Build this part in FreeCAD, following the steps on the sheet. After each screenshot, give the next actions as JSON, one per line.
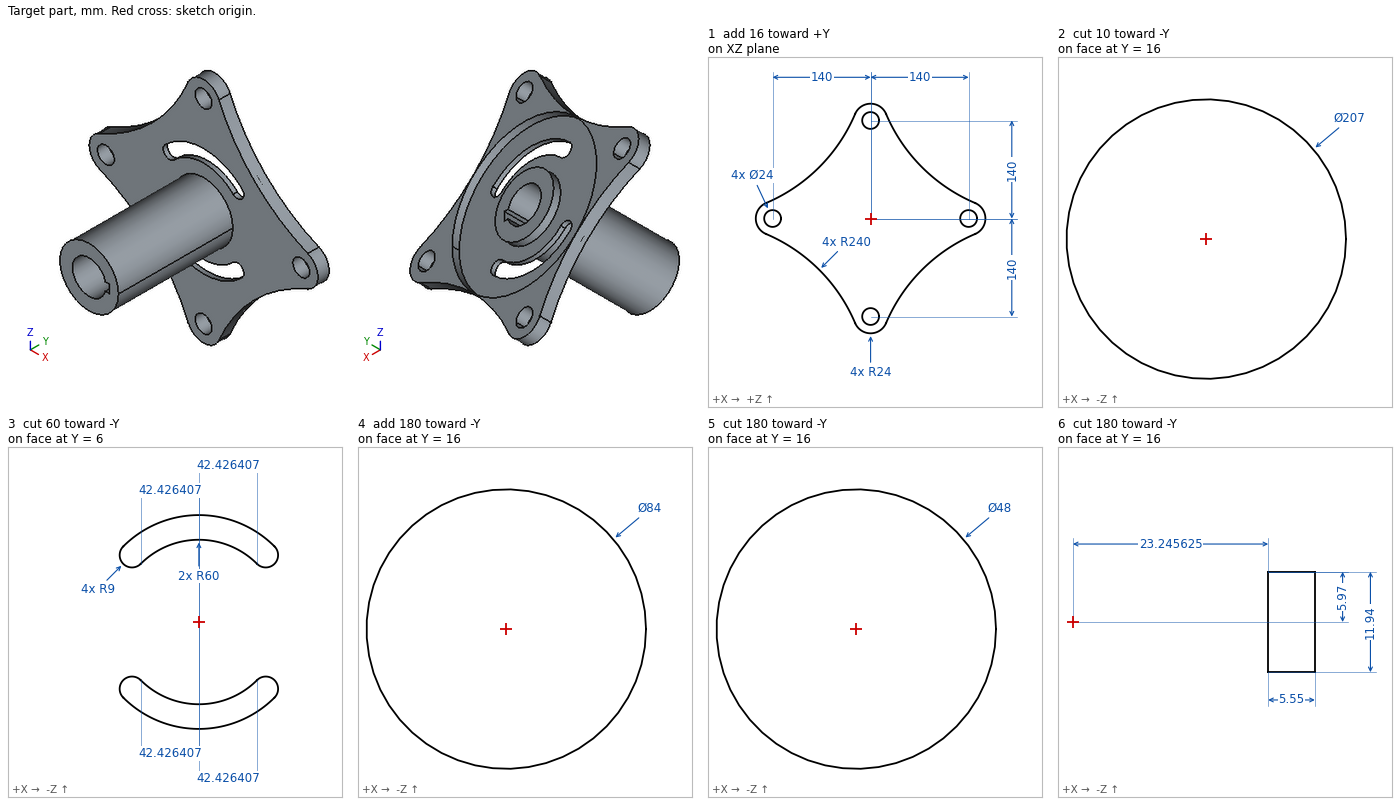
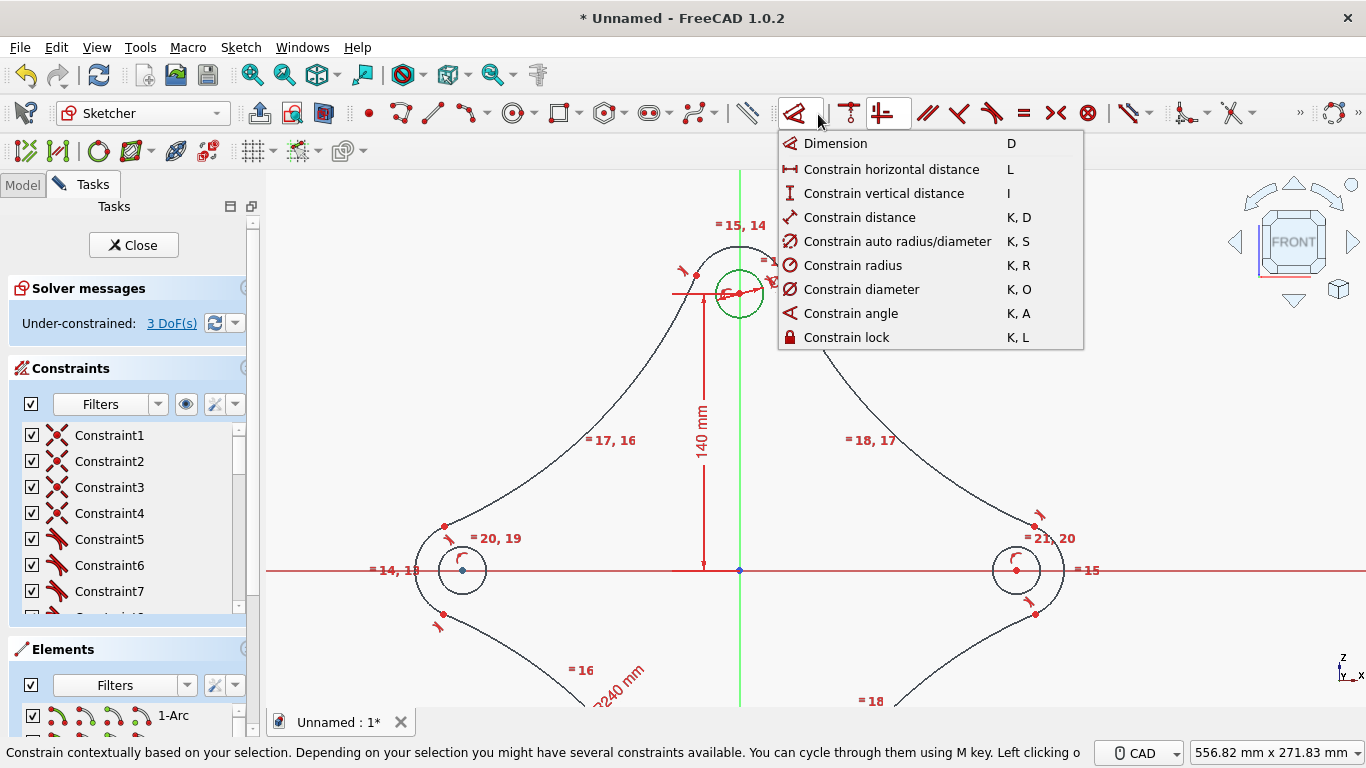
{"action": "left_click", "coordinate": [931, 169]}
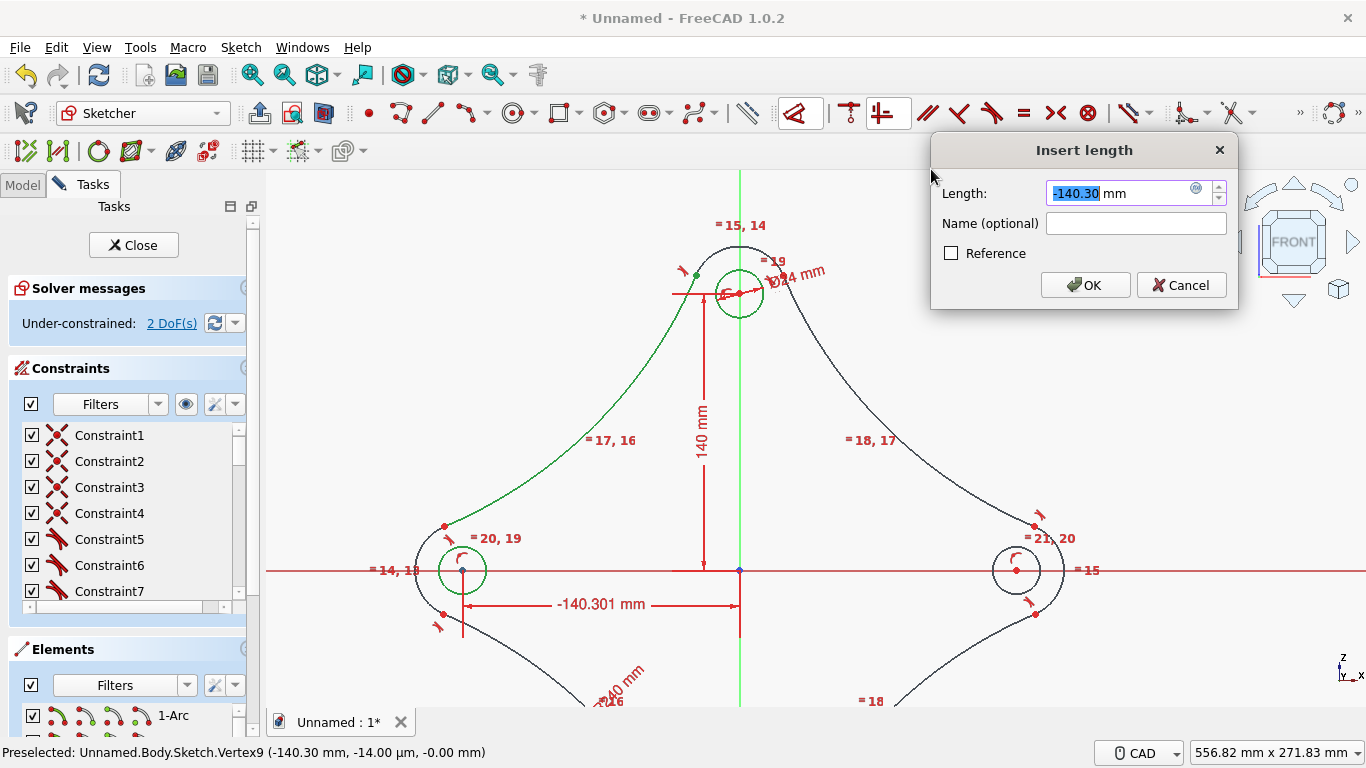
{"action": "type", "text": "-140"}
{"action": "key", "text": "Return"}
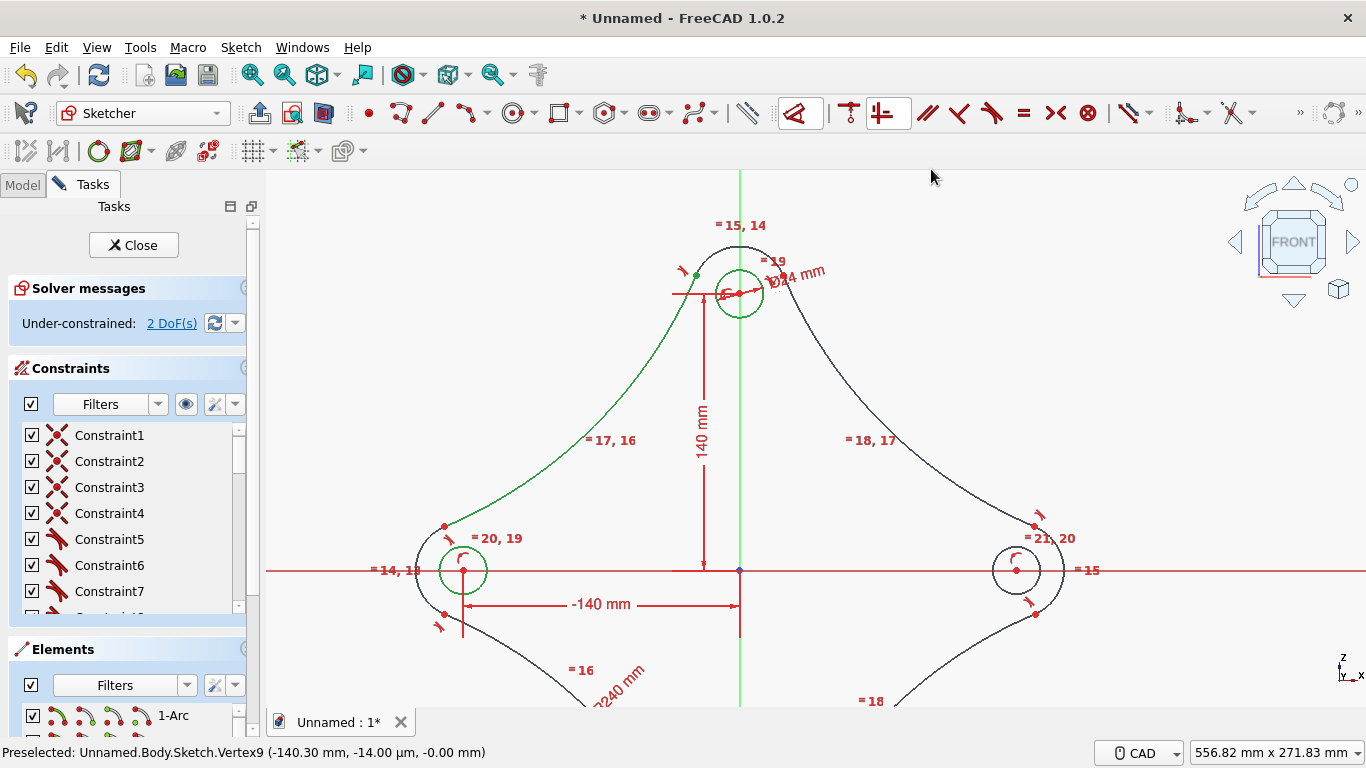
{"action": "left_click", "coordinate": [1016, 571]}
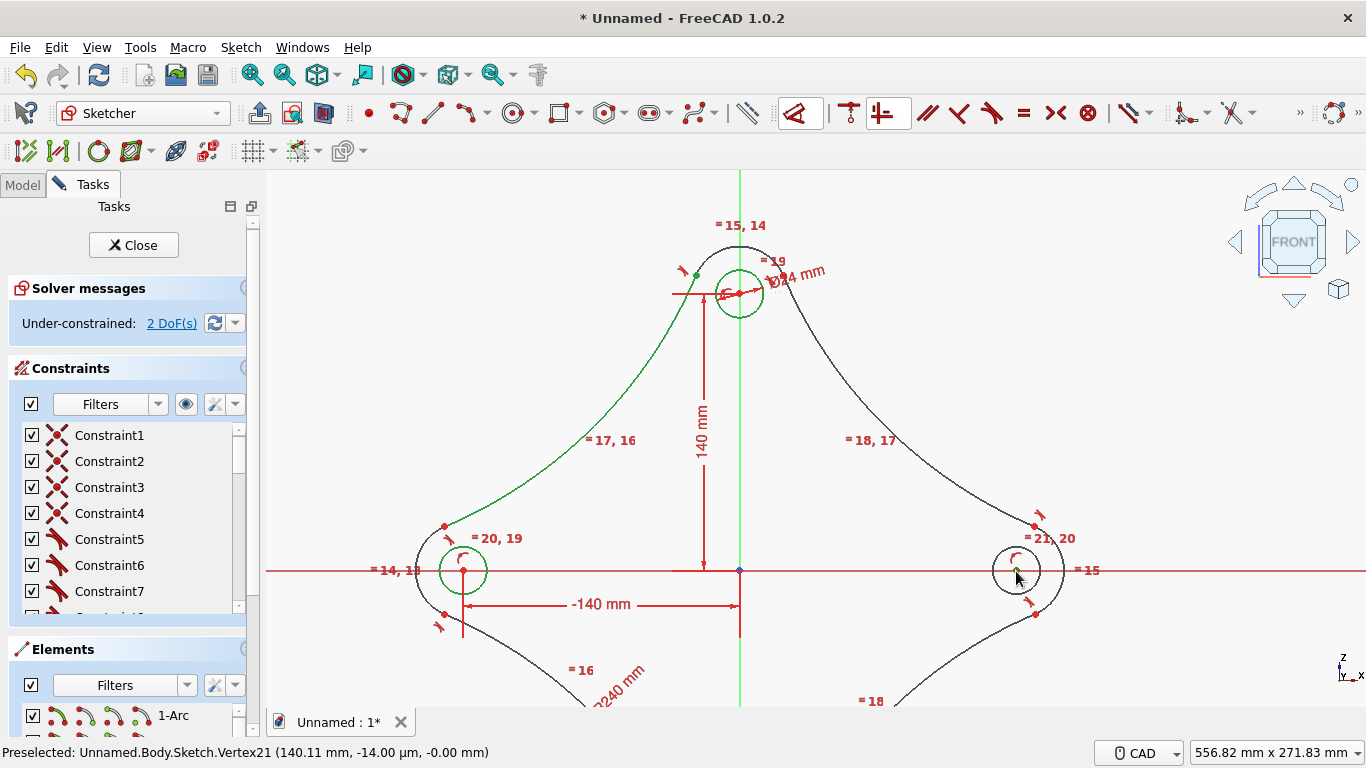
{"action": "left_click", "coordinate": [818, 114]}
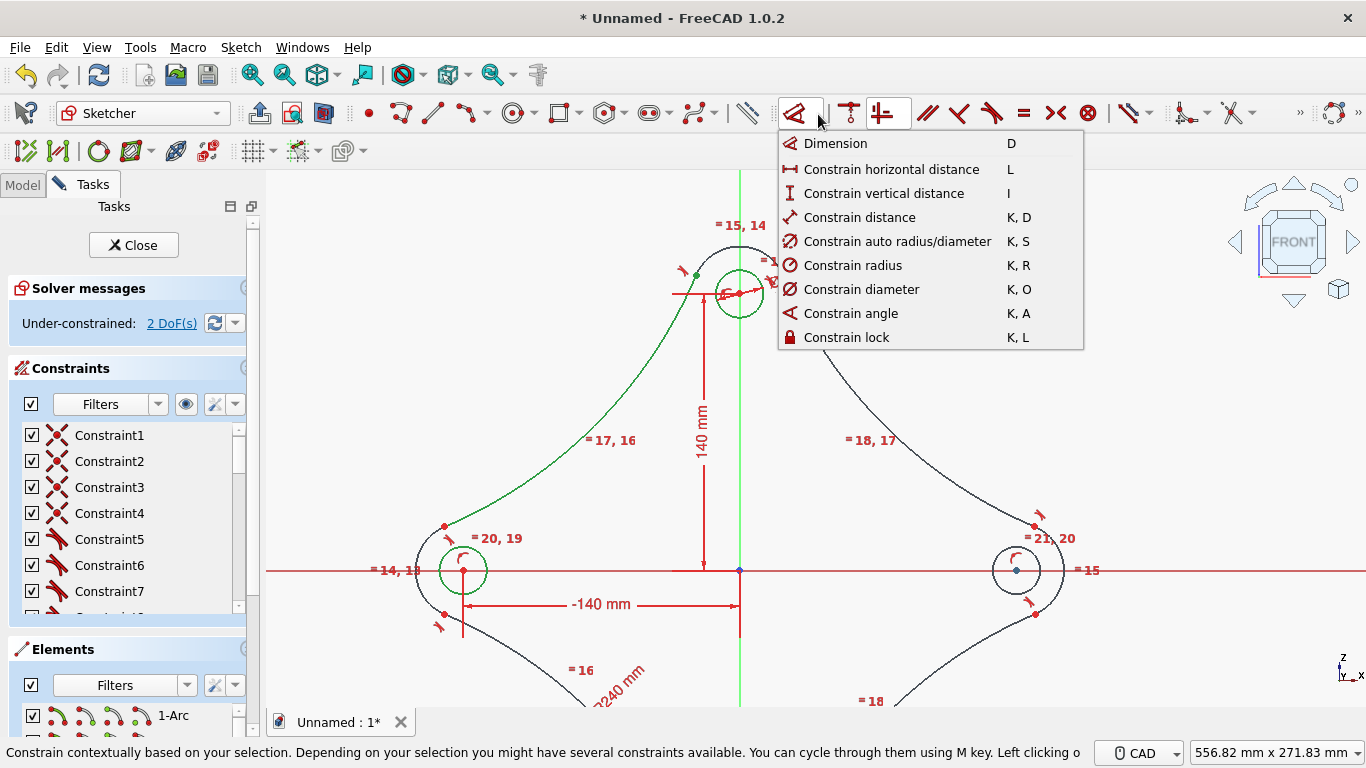
{"action": "left_click", "coordinate": [931, 169]}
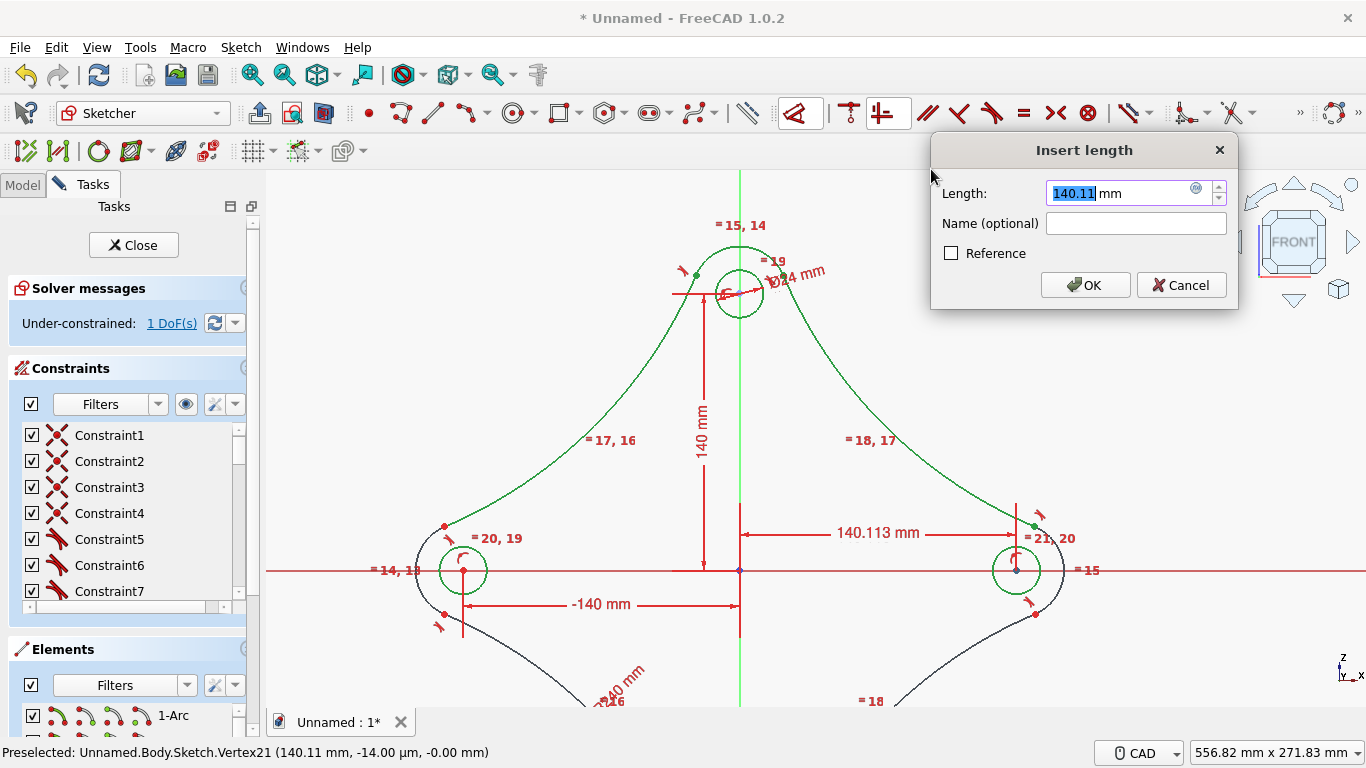
{"action": "type", "text": "140"}
{"action": "key", "text": "Return"}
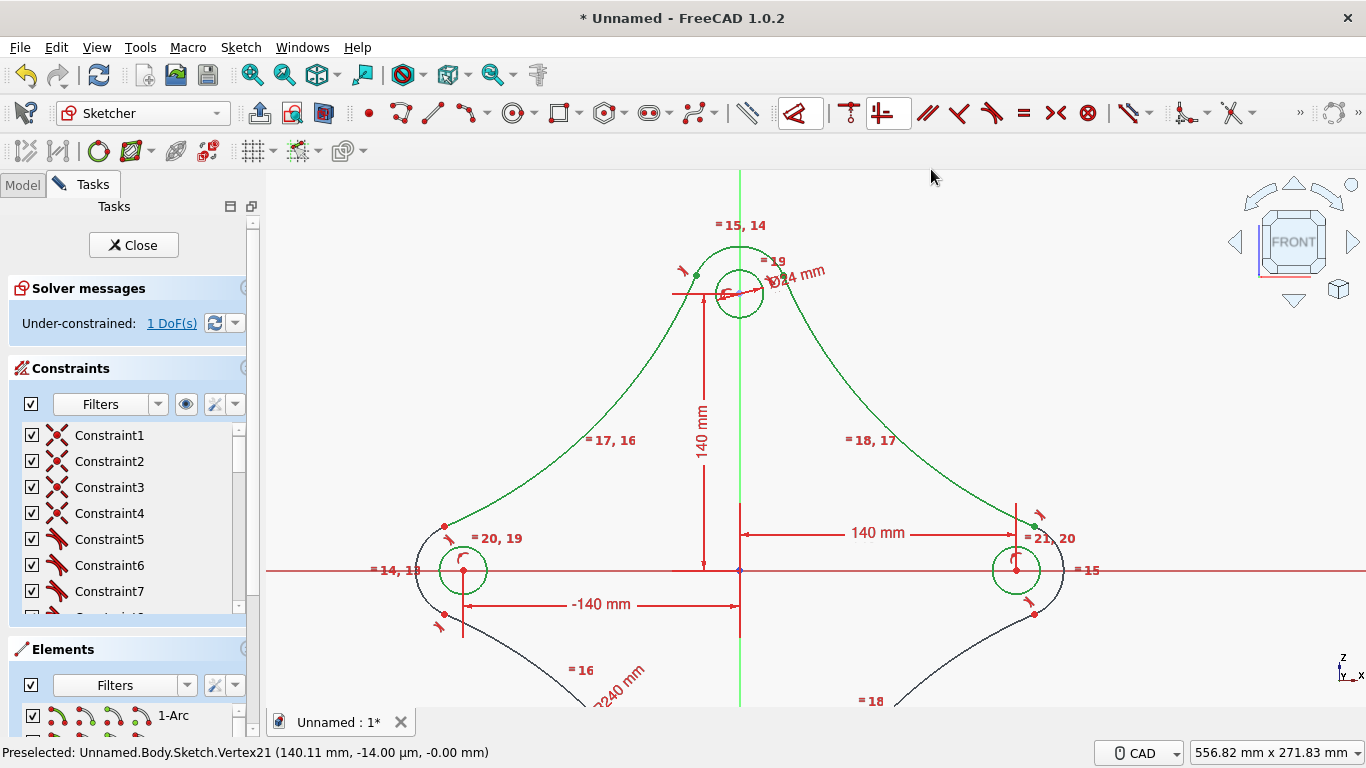
{"action": "scroll", "coordinate": [757, 278], "scroll_direction": "down", "scroll_amount": 3}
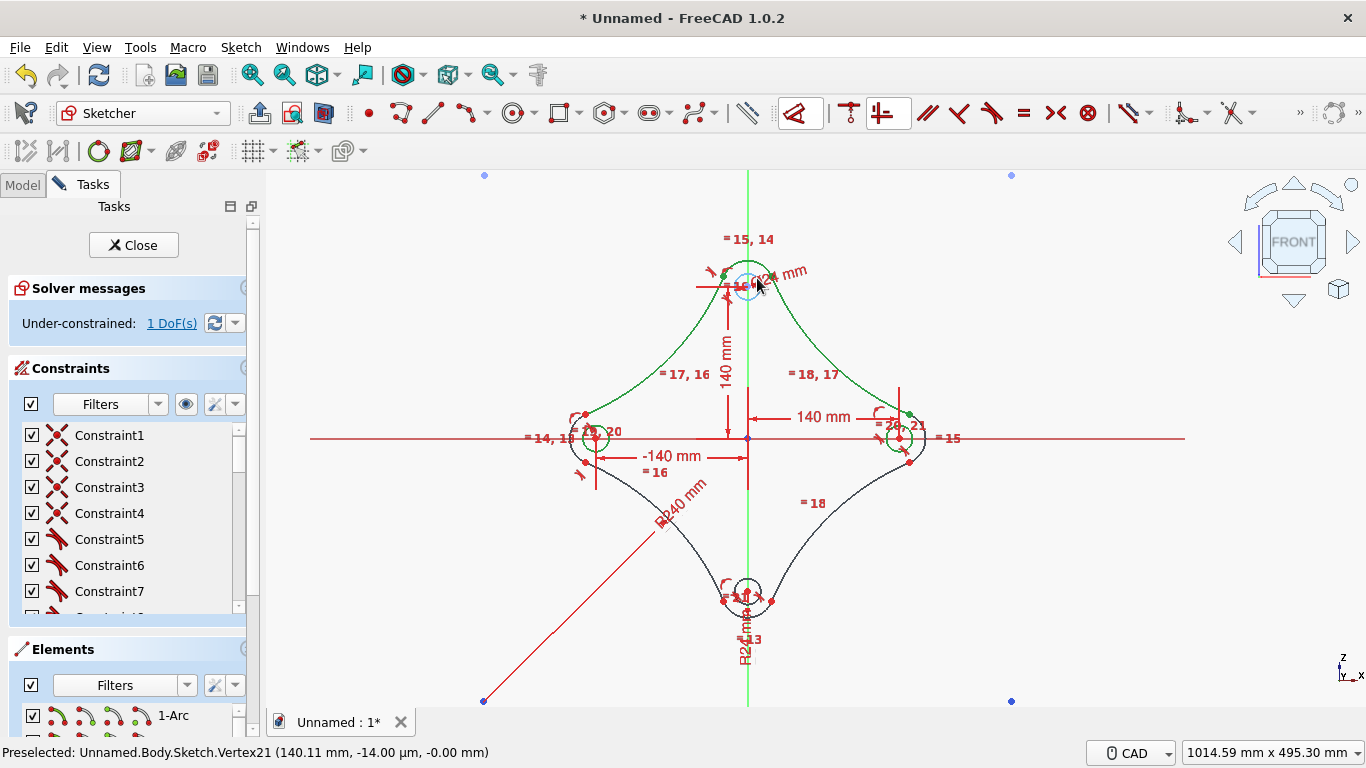
{"action": "left_click", "coordinate": [748, 592]}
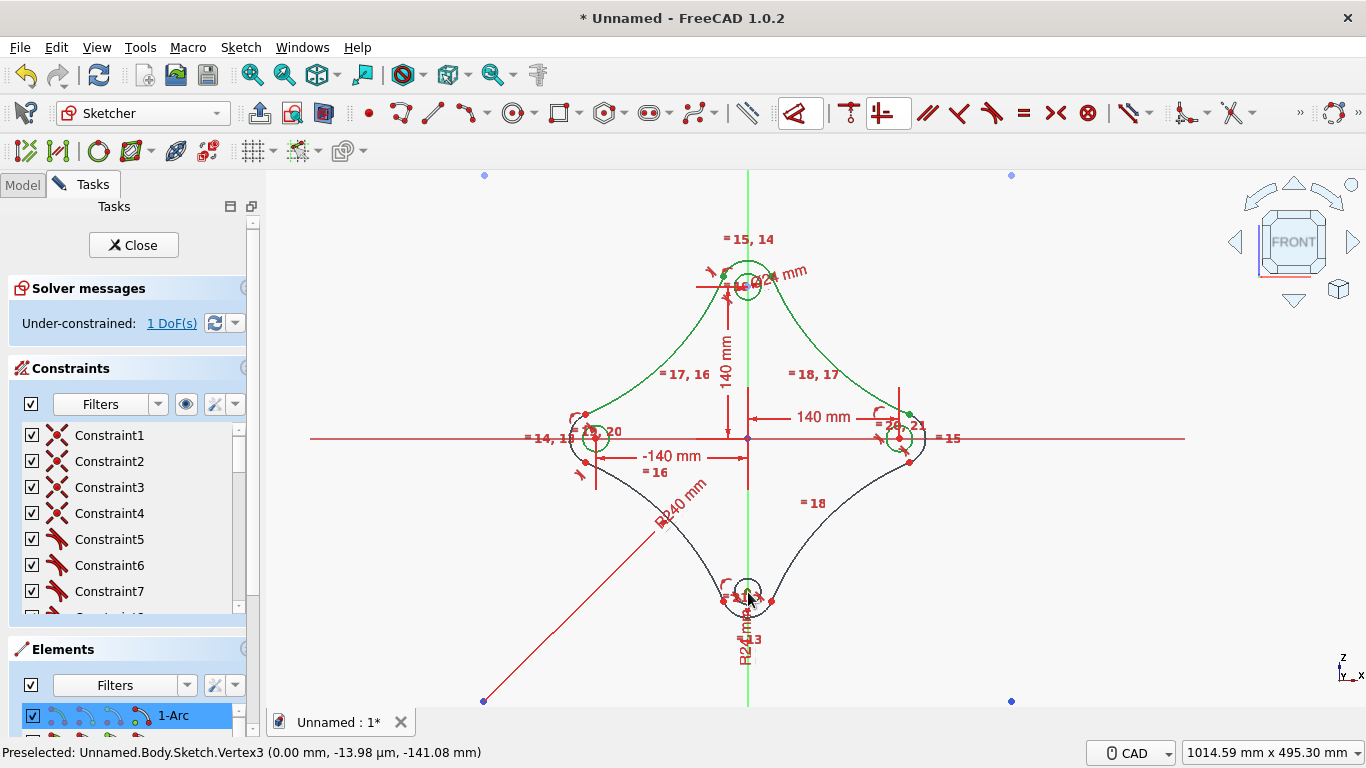
{"action": "key", "text": "i"}